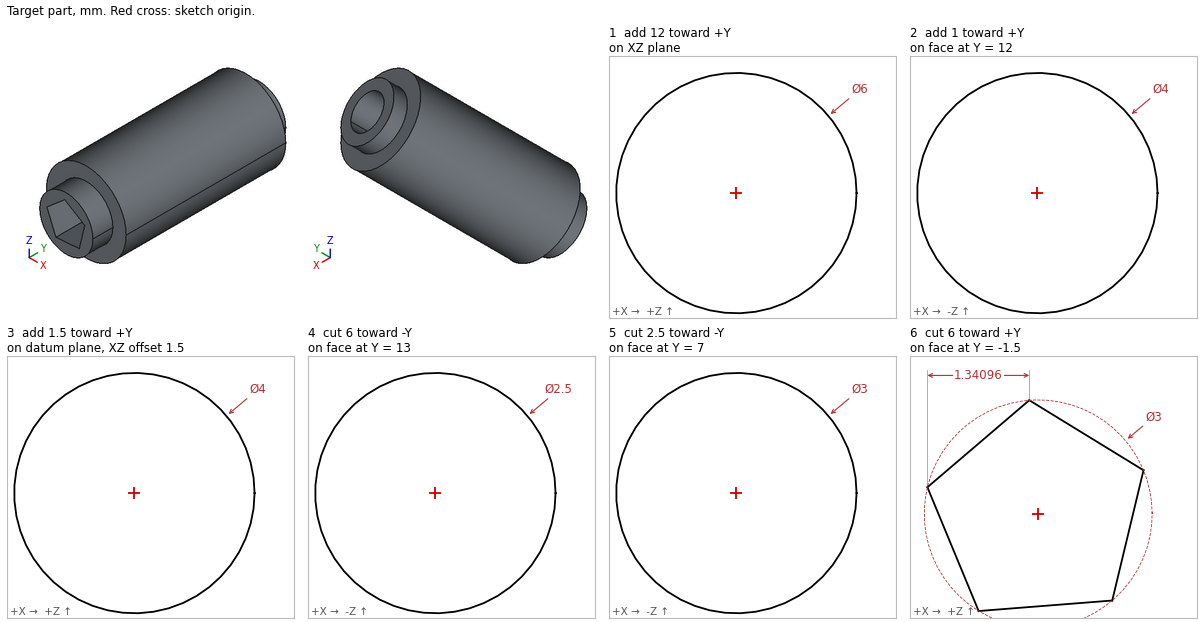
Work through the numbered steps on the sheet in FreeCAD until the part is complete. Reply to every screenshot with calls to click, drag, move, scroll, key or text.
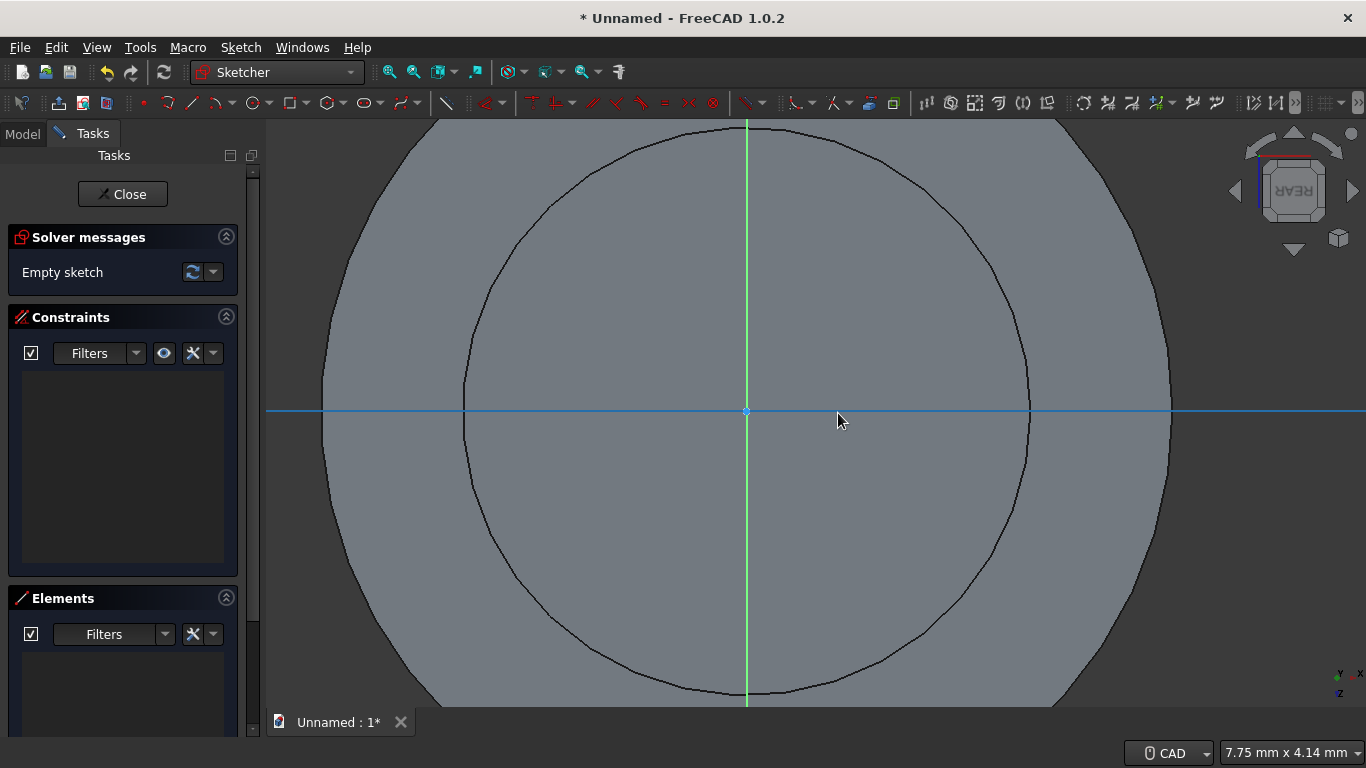
click(254, 104)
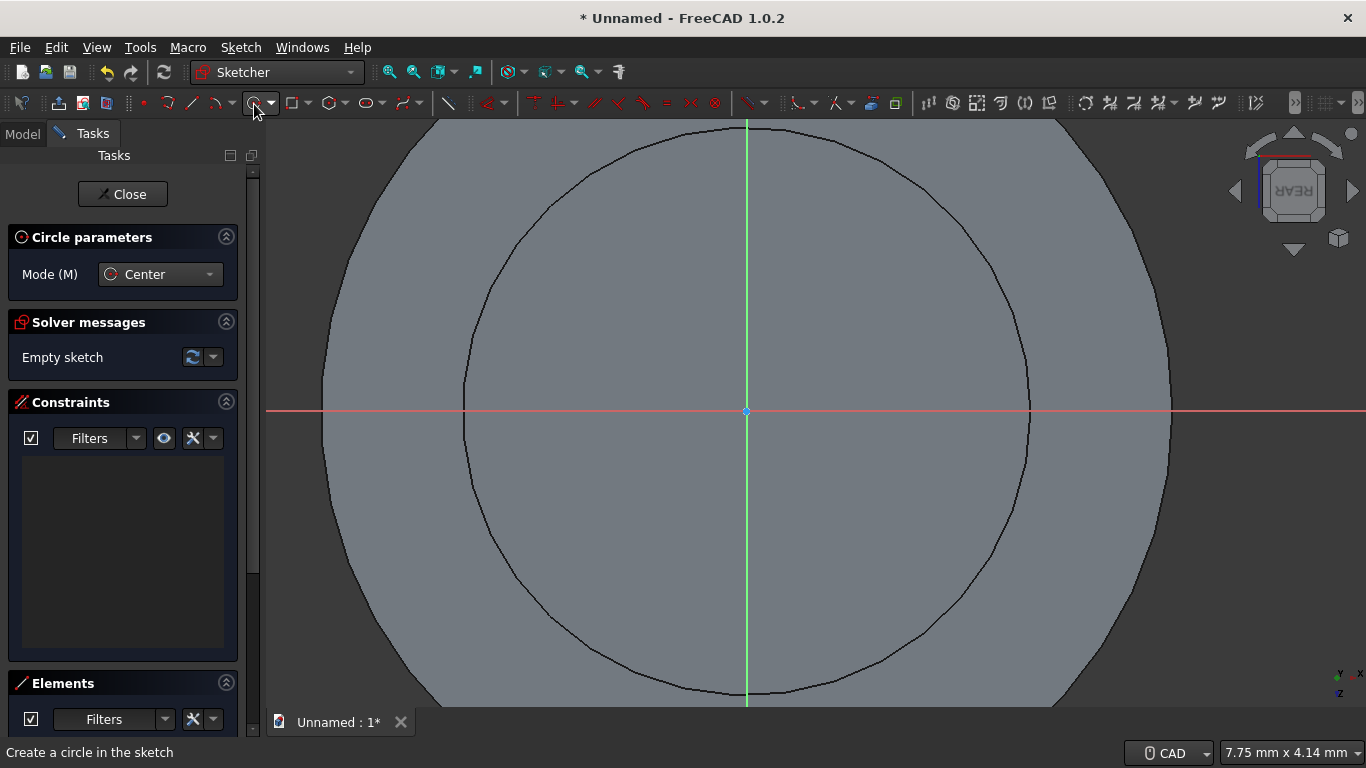
click(747, 411)
move(872, 286)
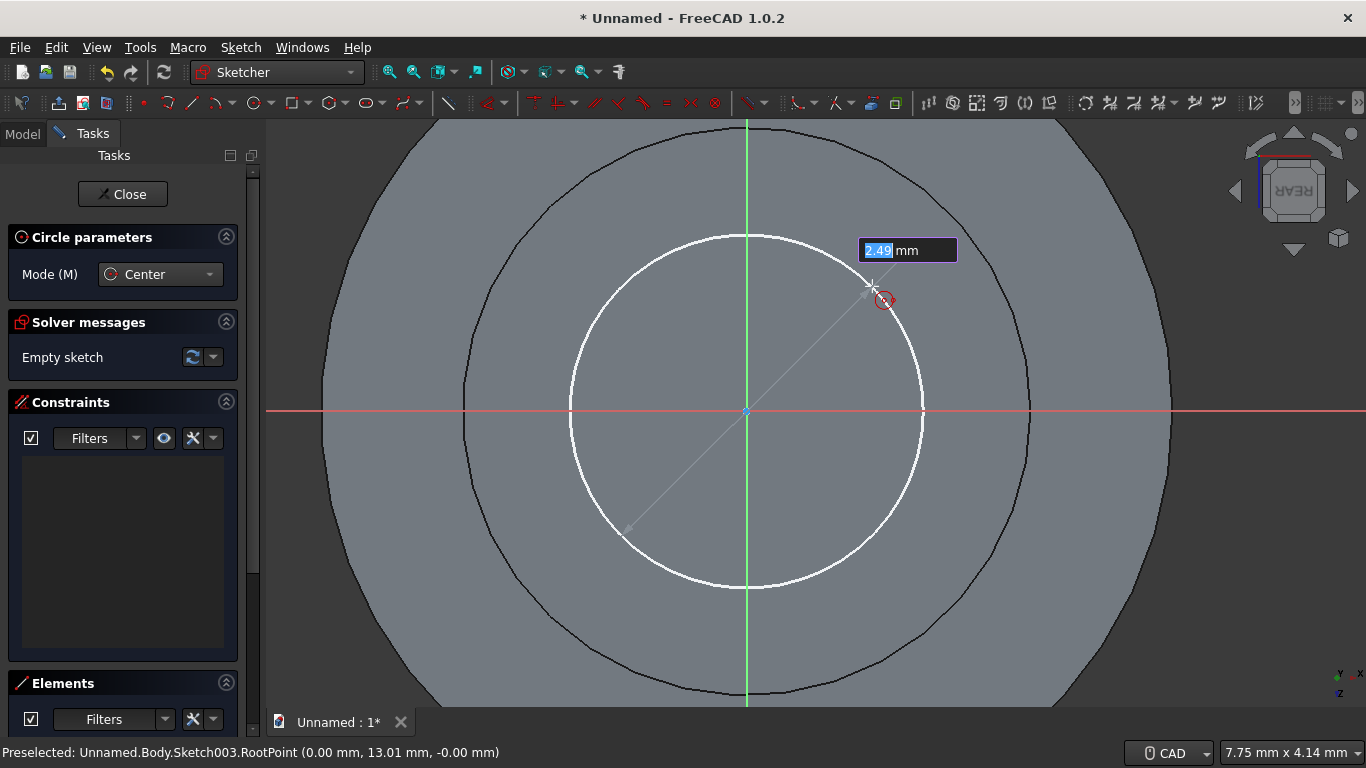
text(2.5)
key(Return)
key(Escape)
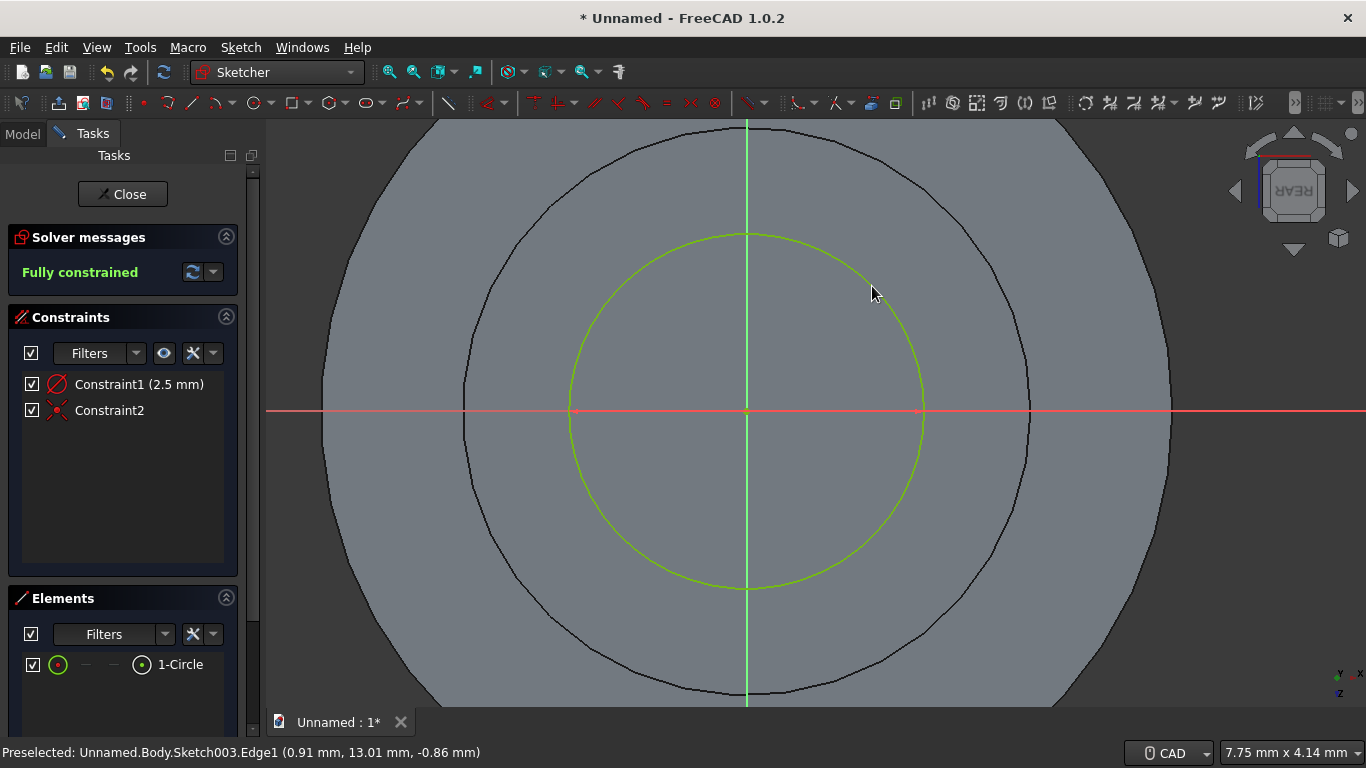
click(123, 194)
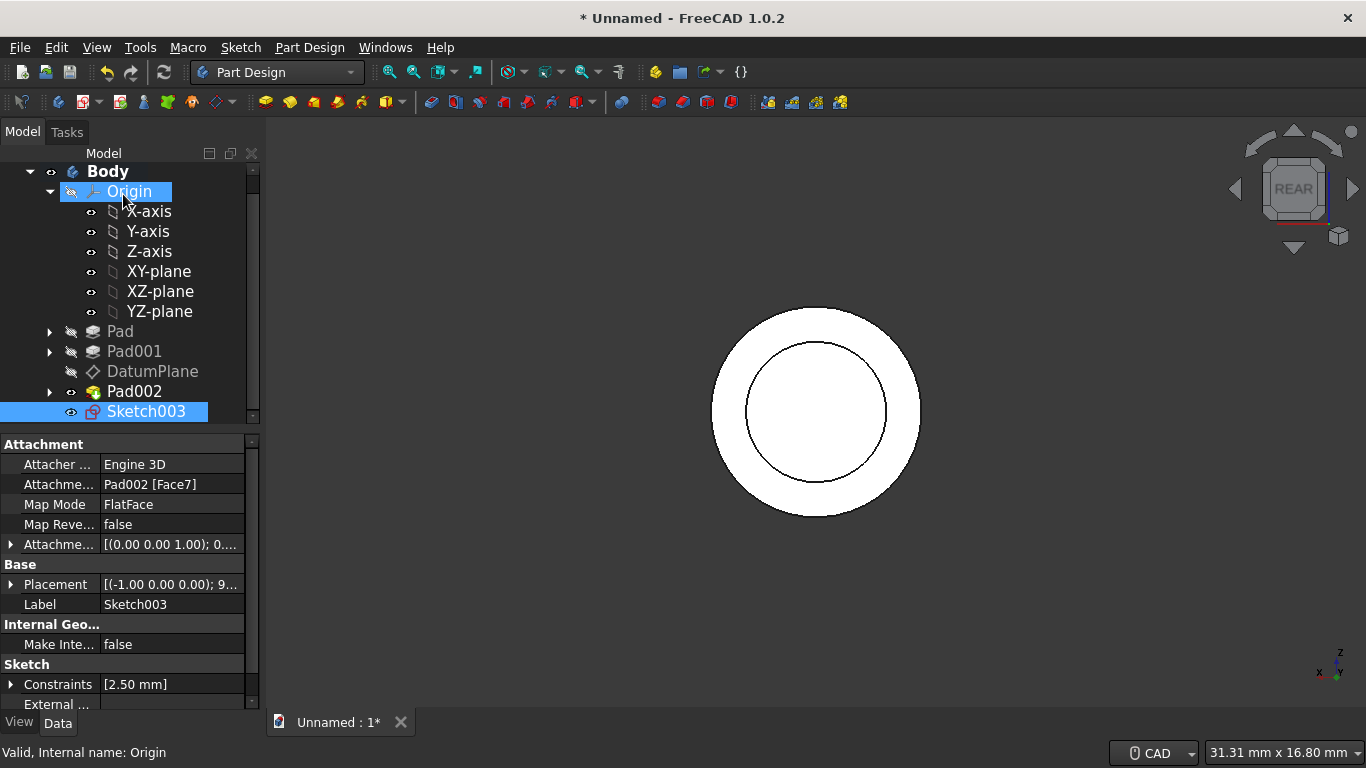
click(432, 102)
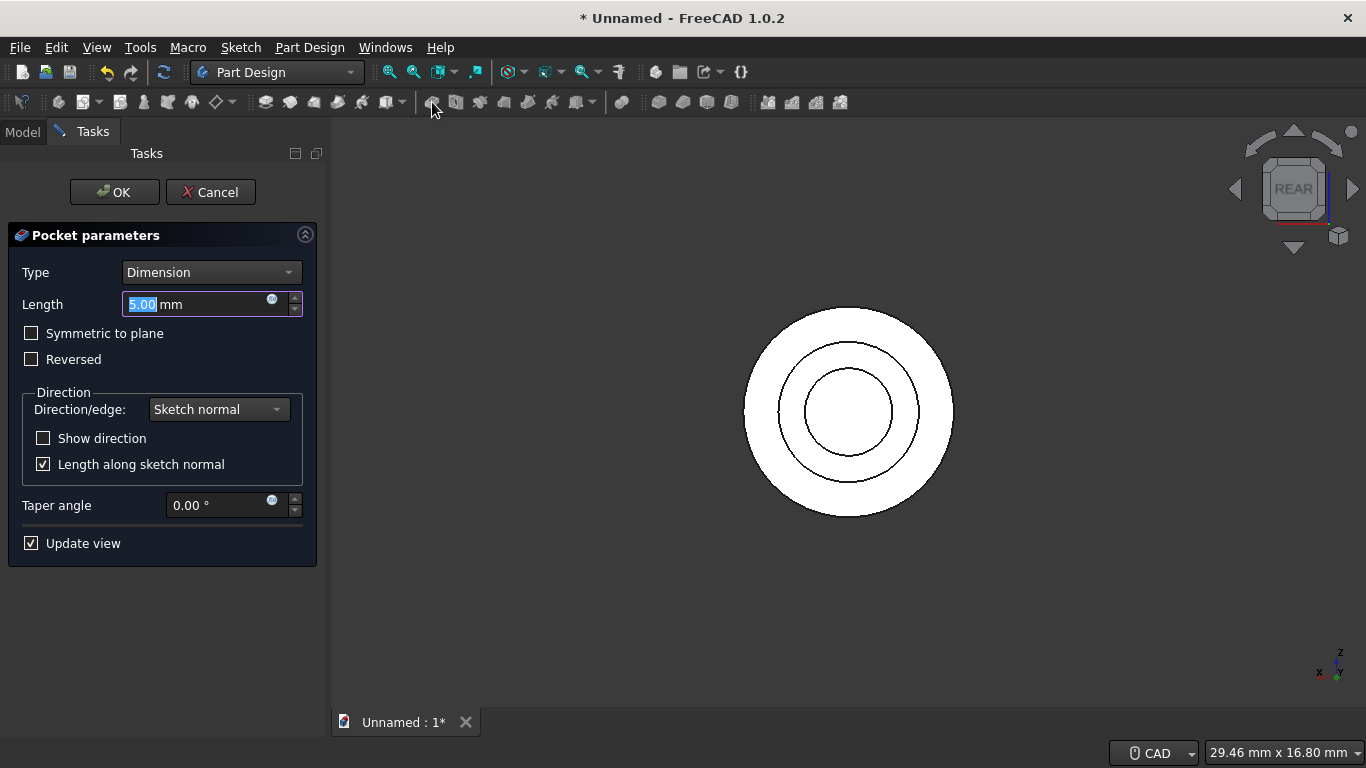
text(6)
key(Tab)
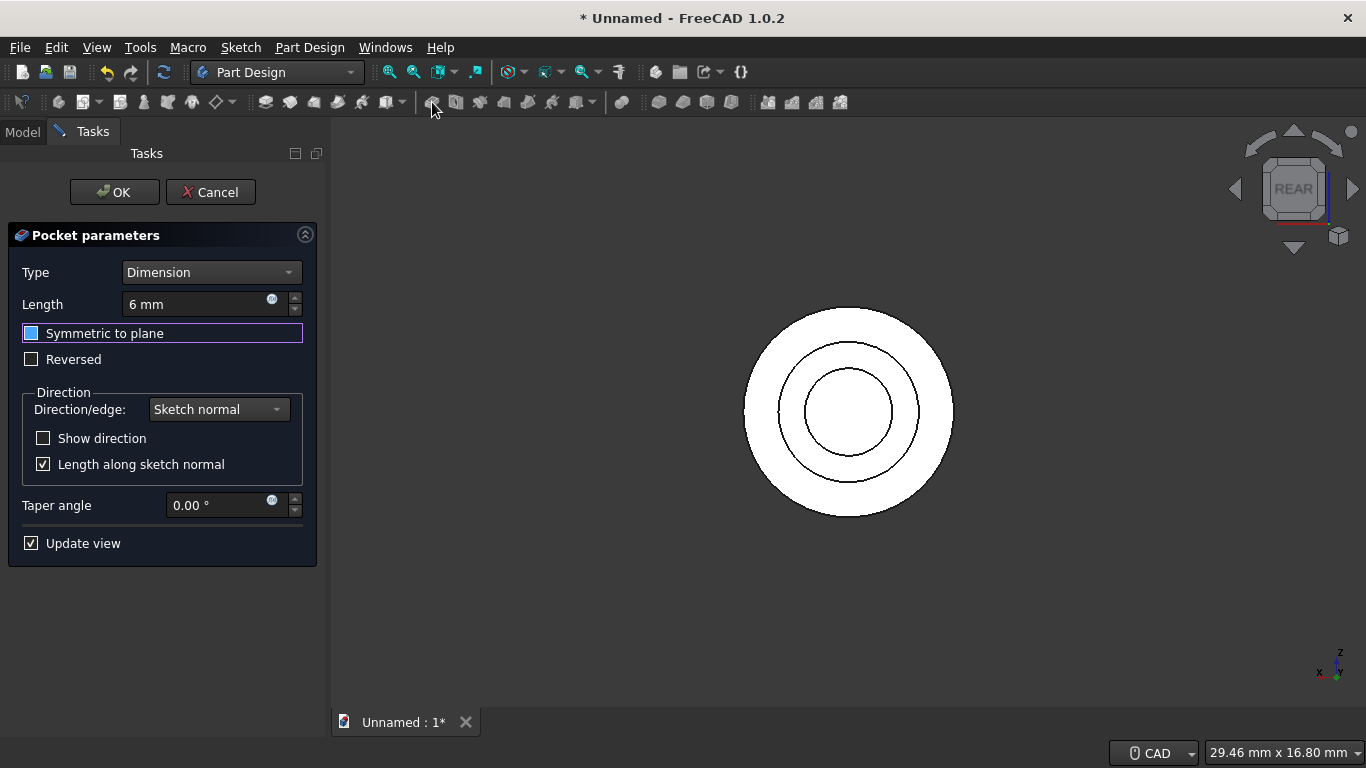
click(115, 192)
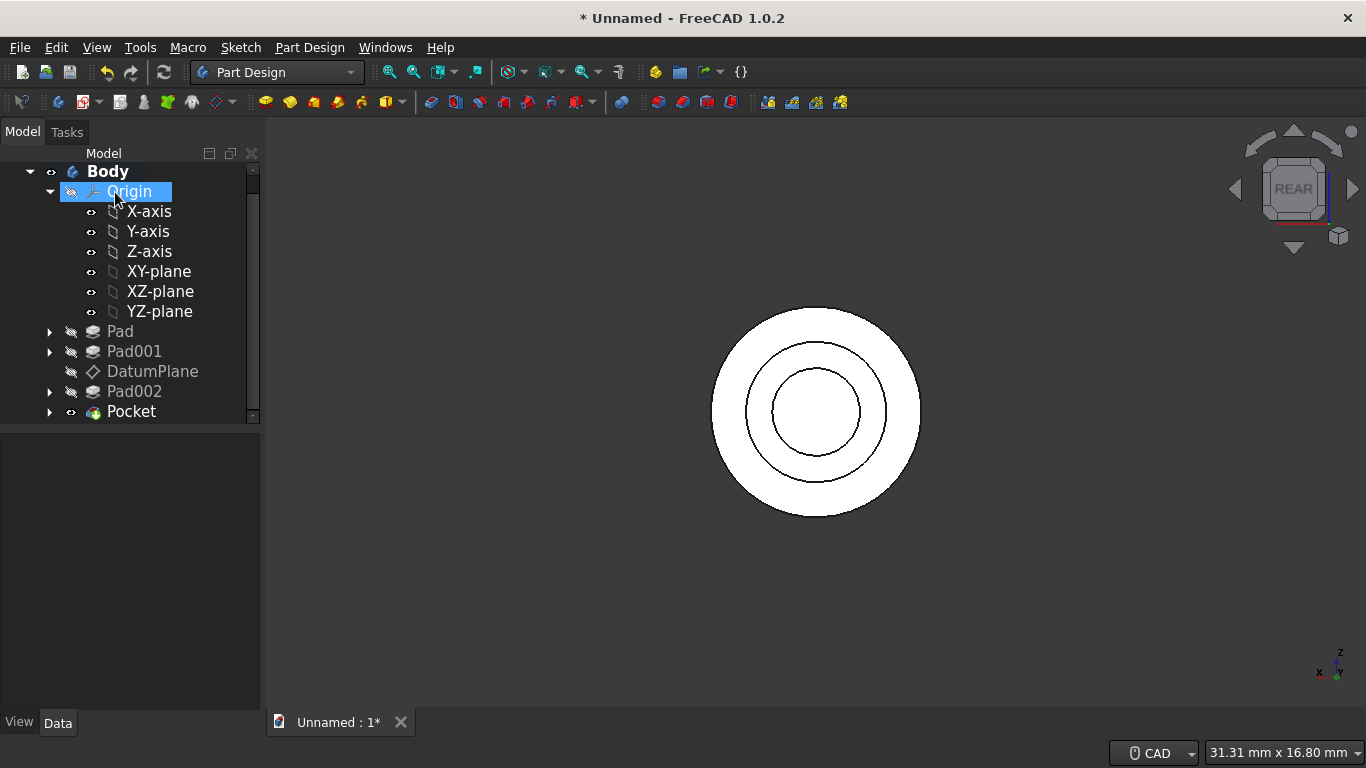
click(390, 72)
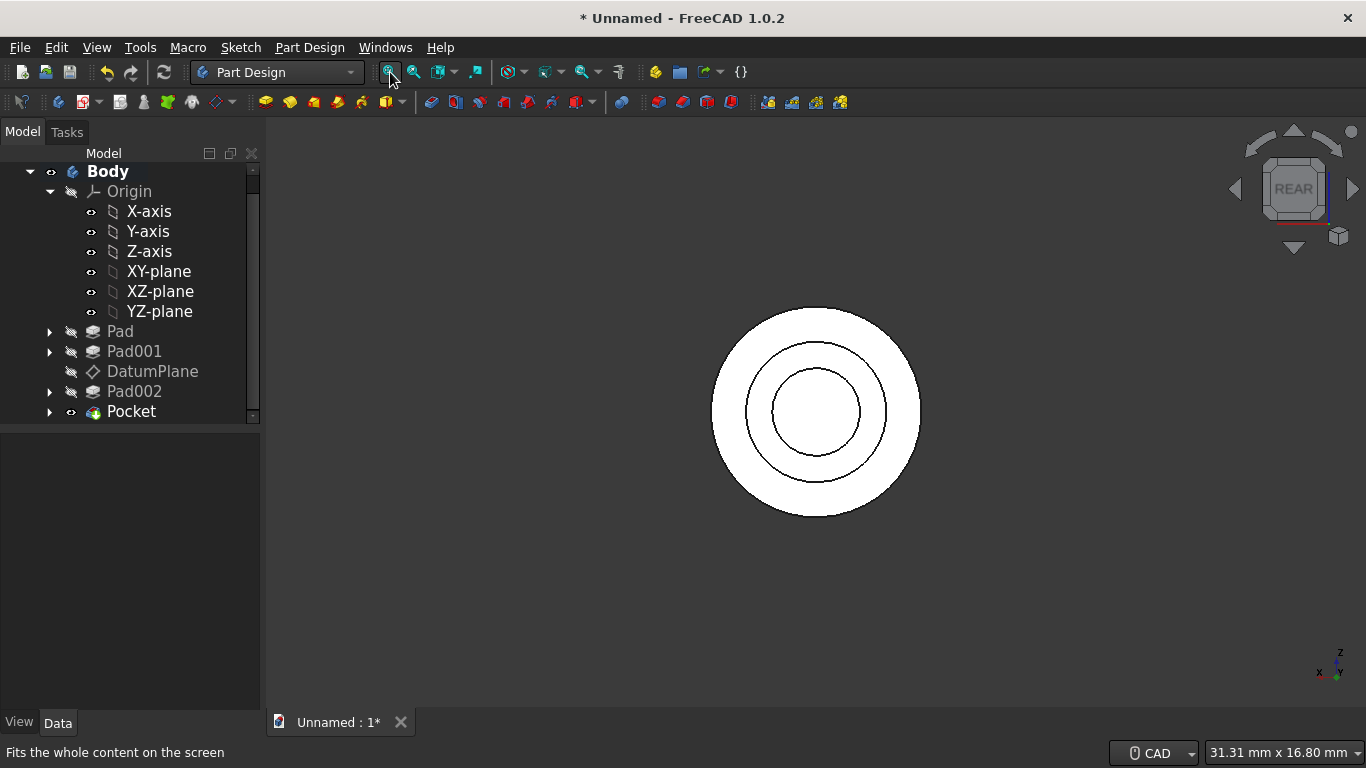
click(816, 411)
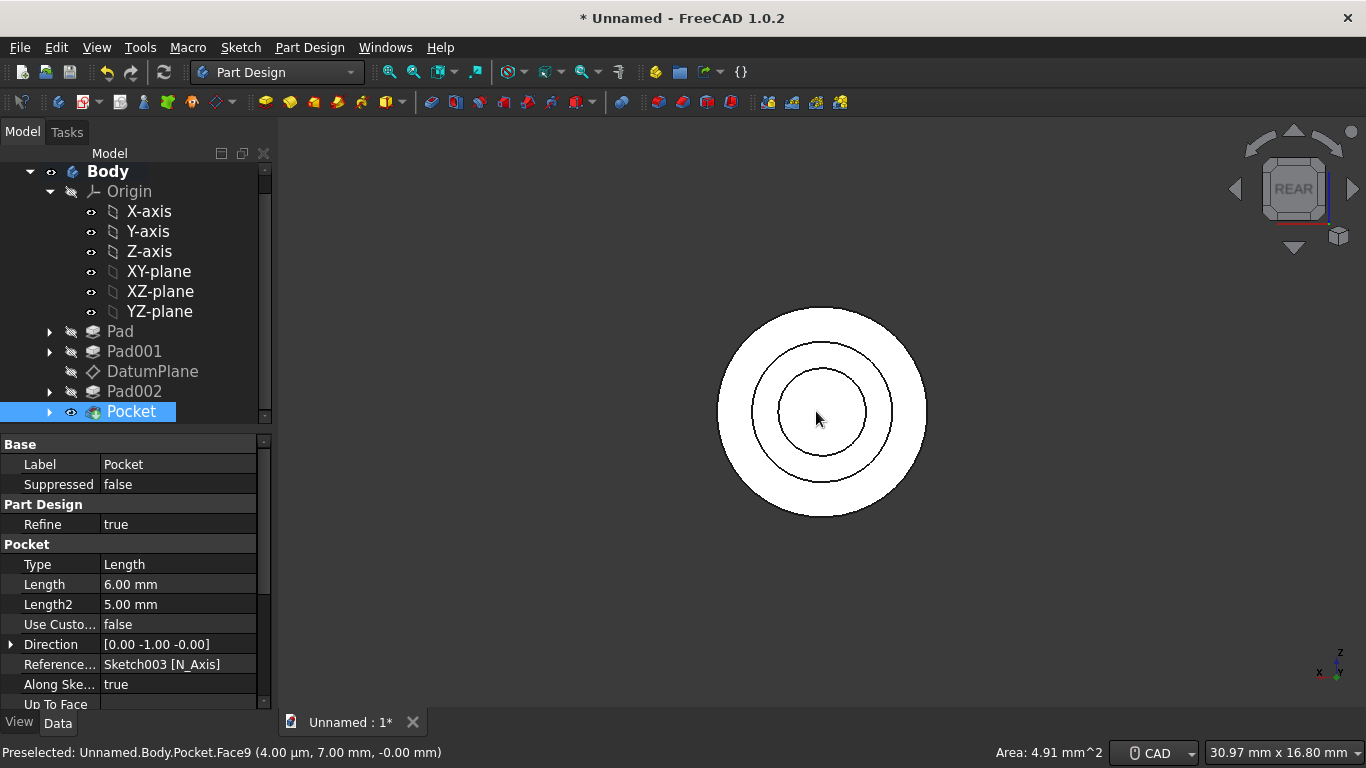
click(84, 102)